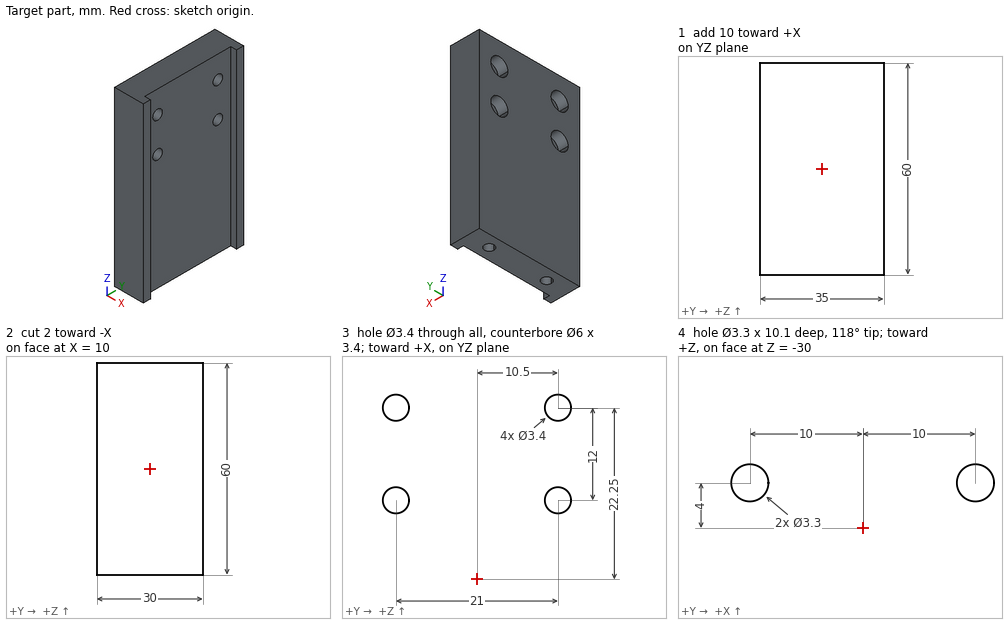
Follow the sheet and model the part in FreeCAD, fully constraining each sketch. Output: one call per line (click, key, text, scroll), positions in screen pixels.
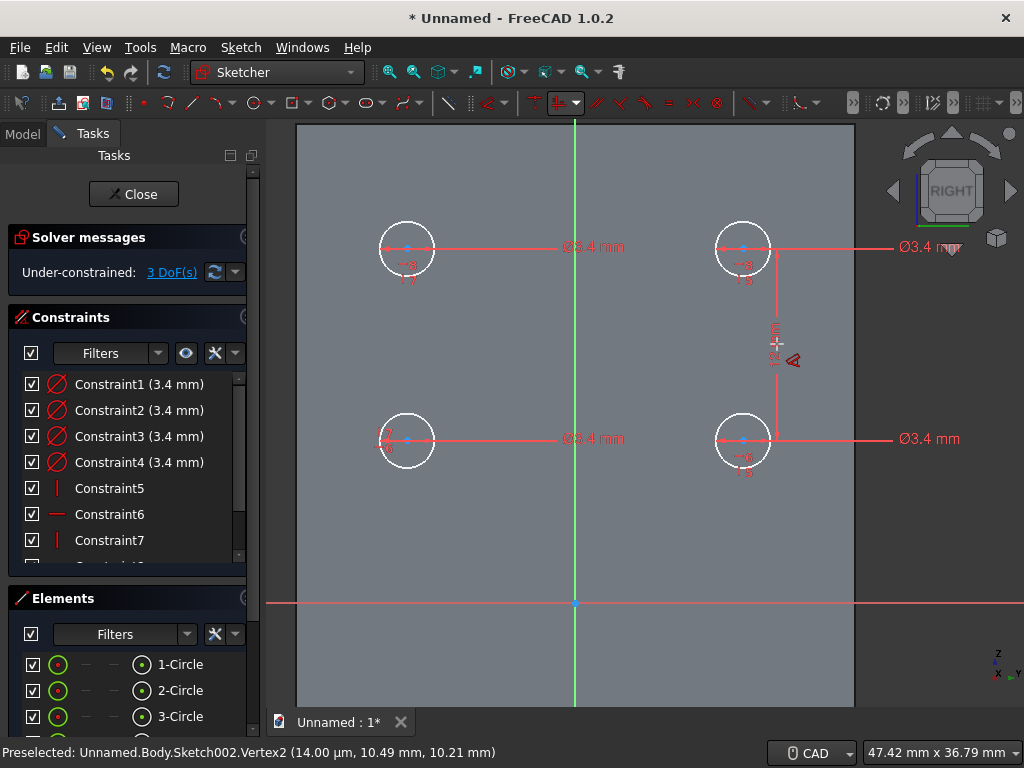
click(743, 441)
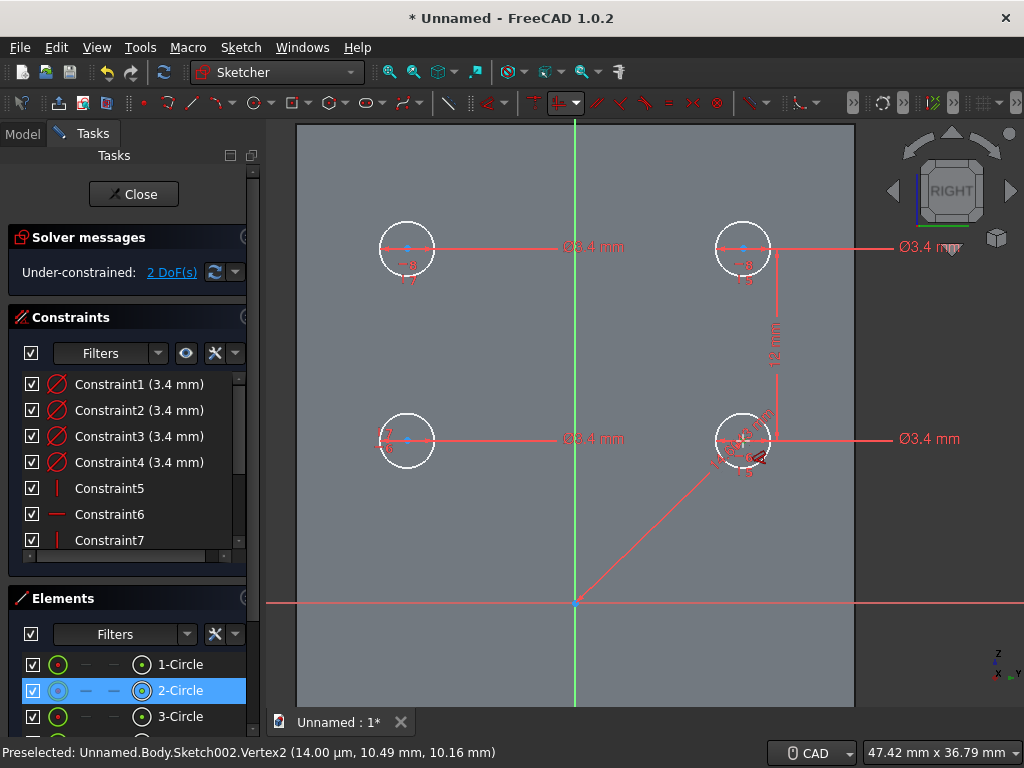
click(407, 441)
click(498, 475)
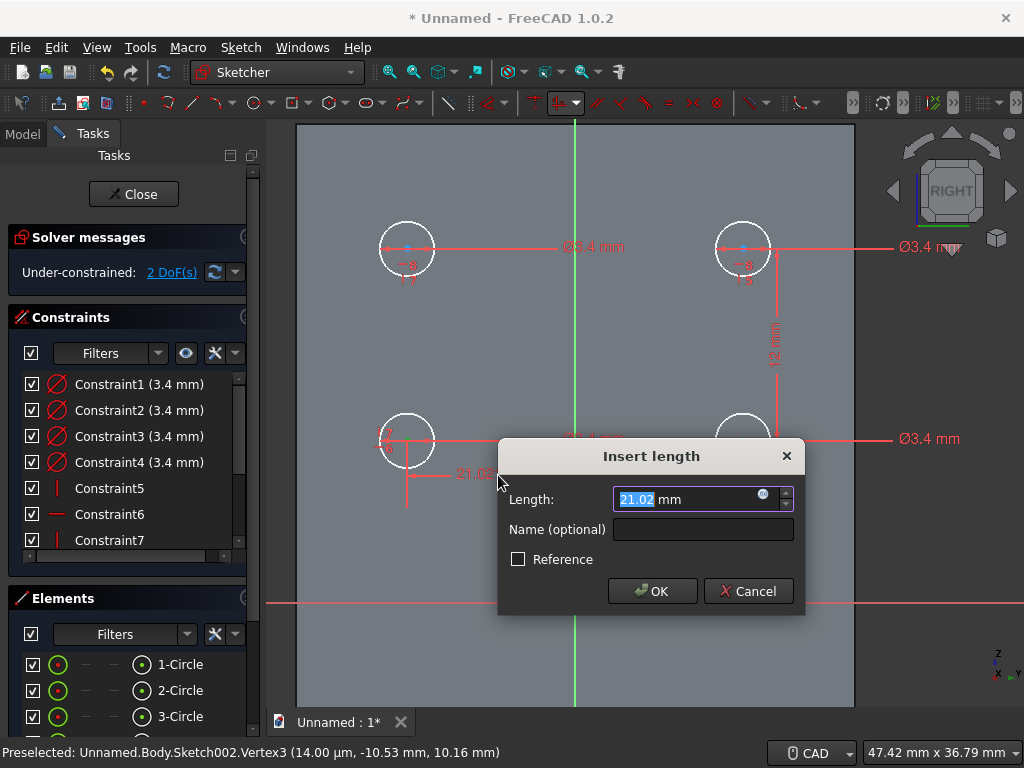
text(21)
key(Return)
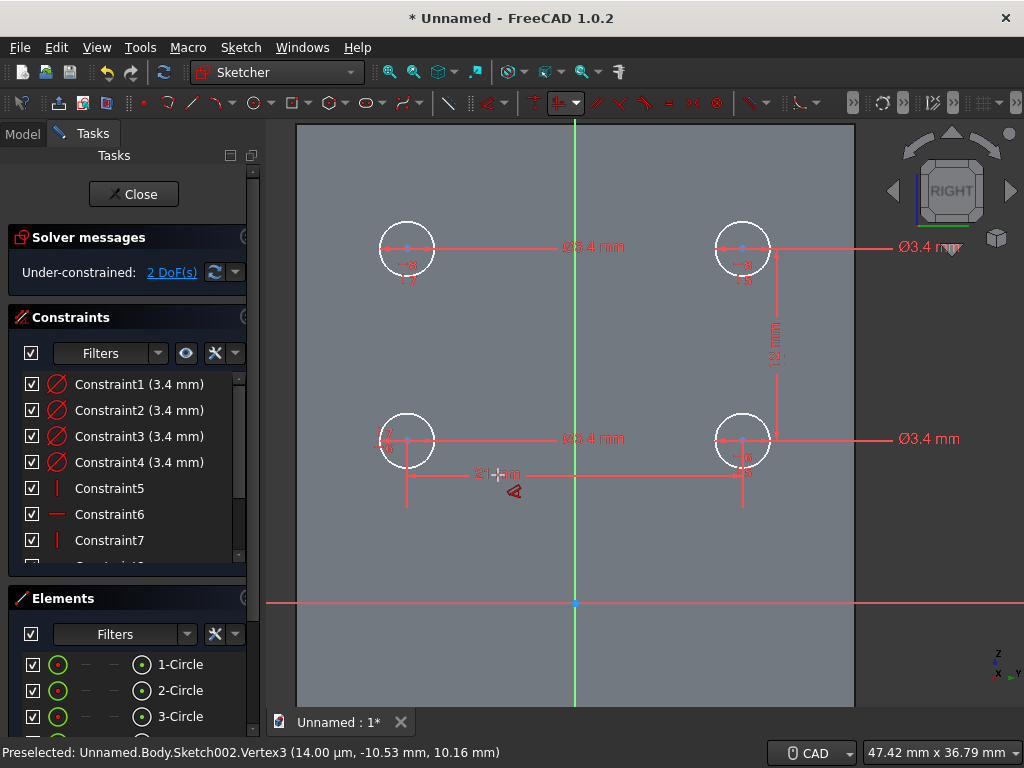
click(743, 249)
click(659, 637)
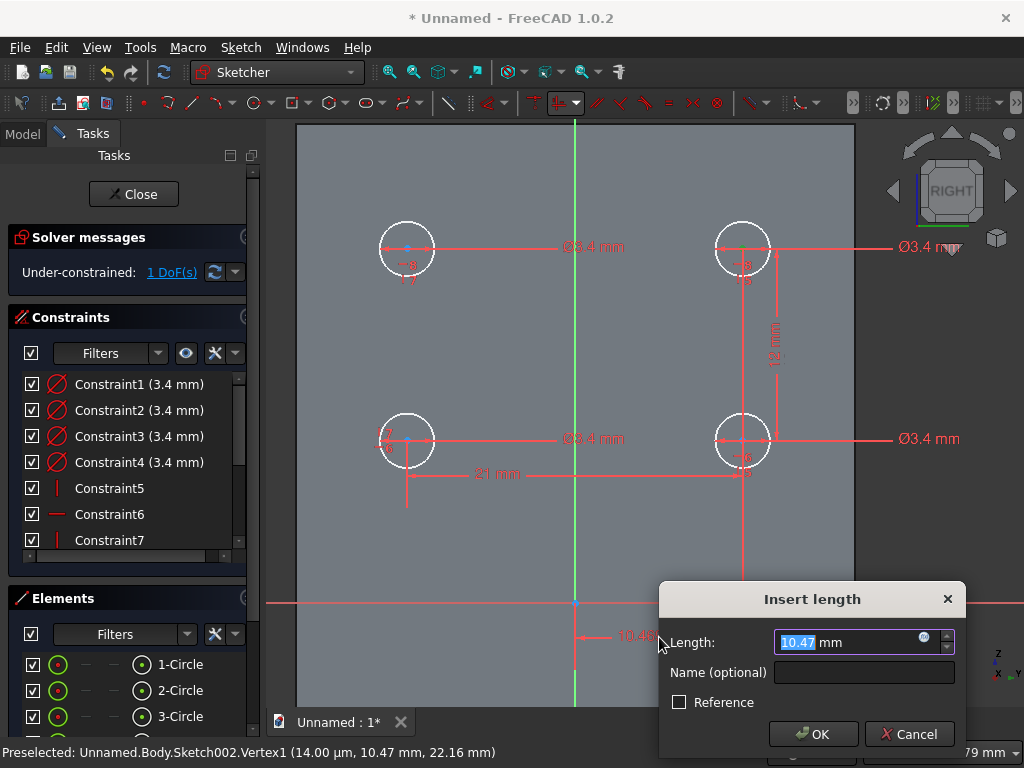
text(10.5)
key(Return)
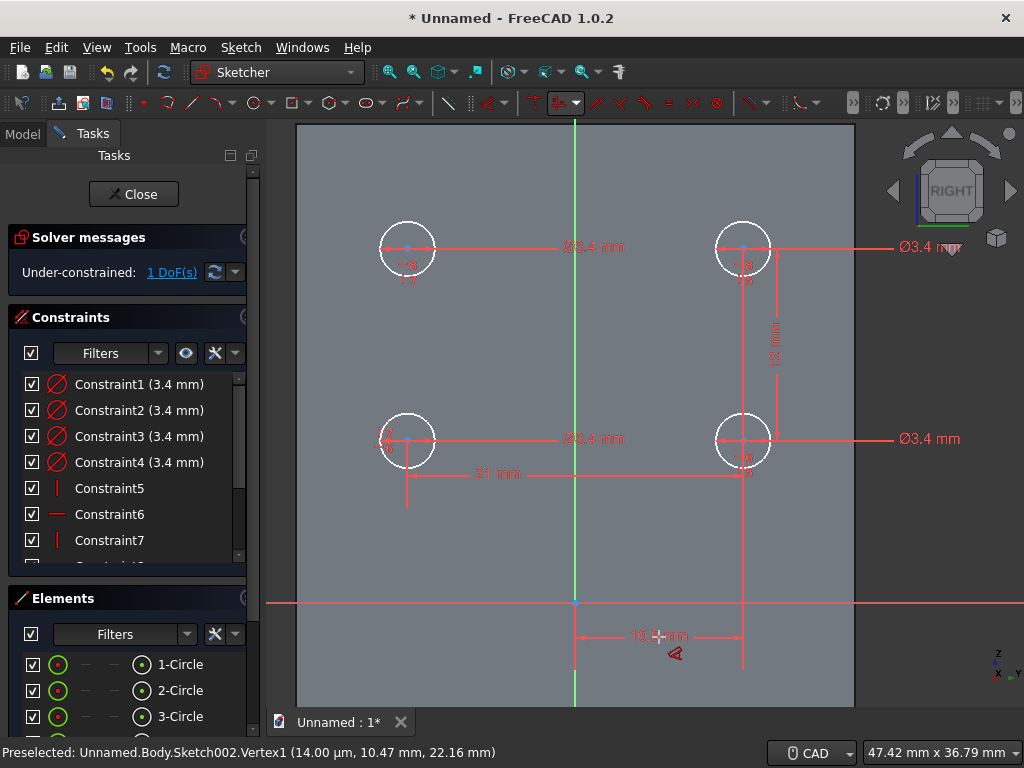
click(743, 249)
click(777, 508)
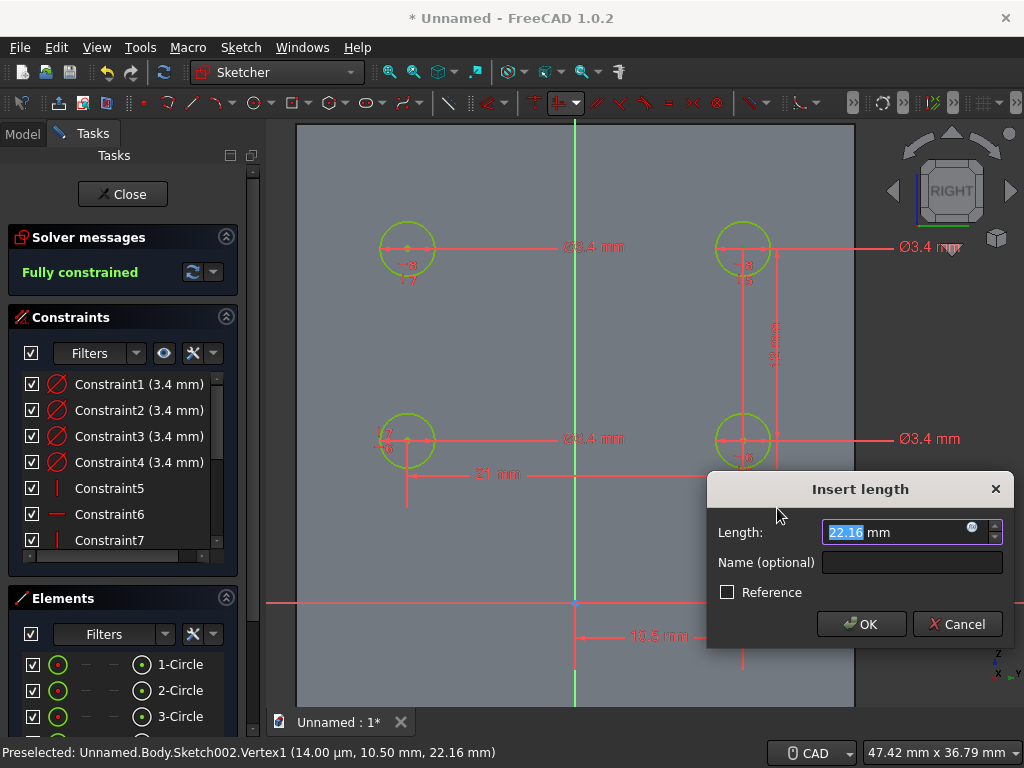
text(22.25)
key(Return)
key(Escape)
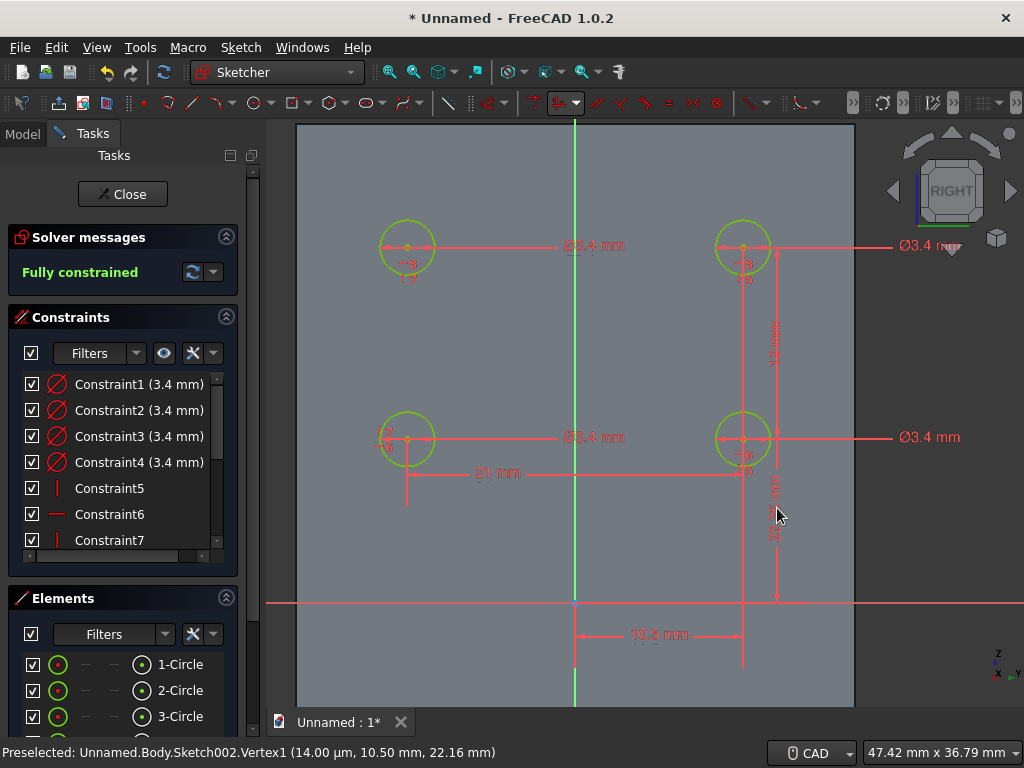
click(123, 194)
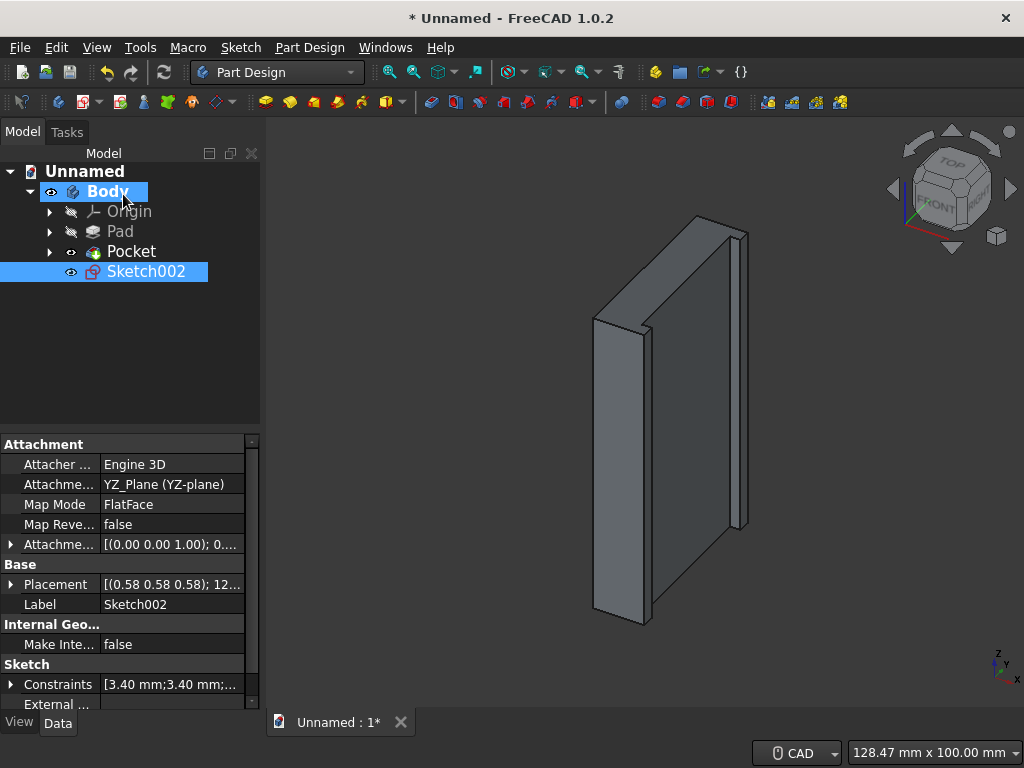
click(456, 102)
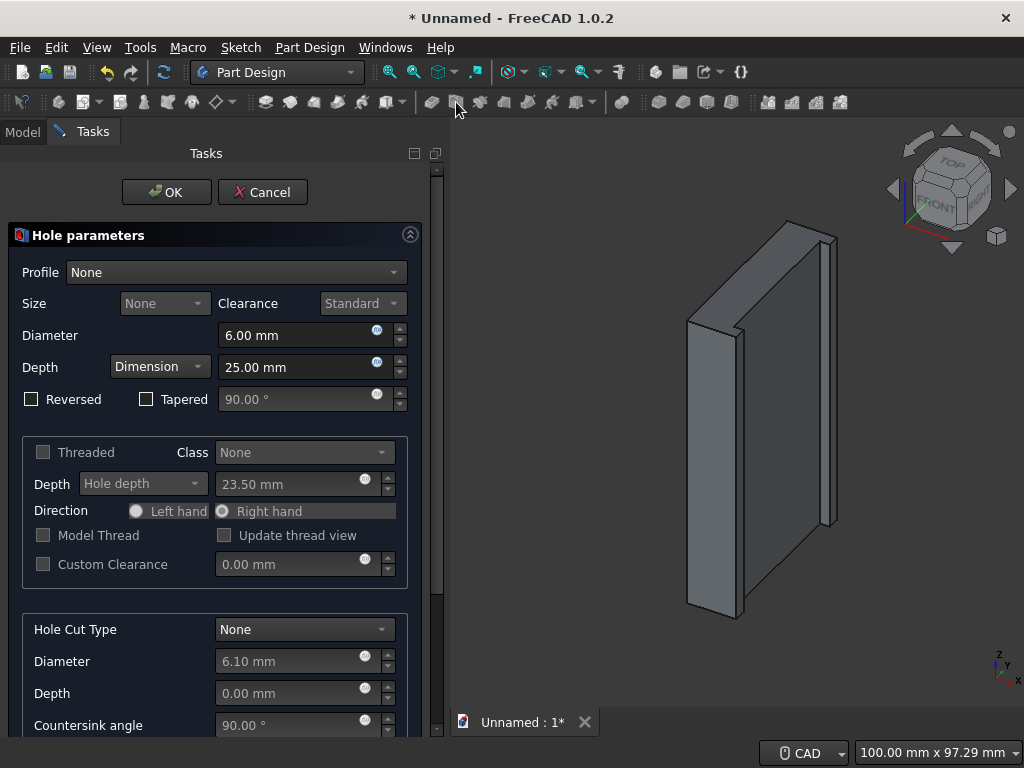
triple_click(305, 335)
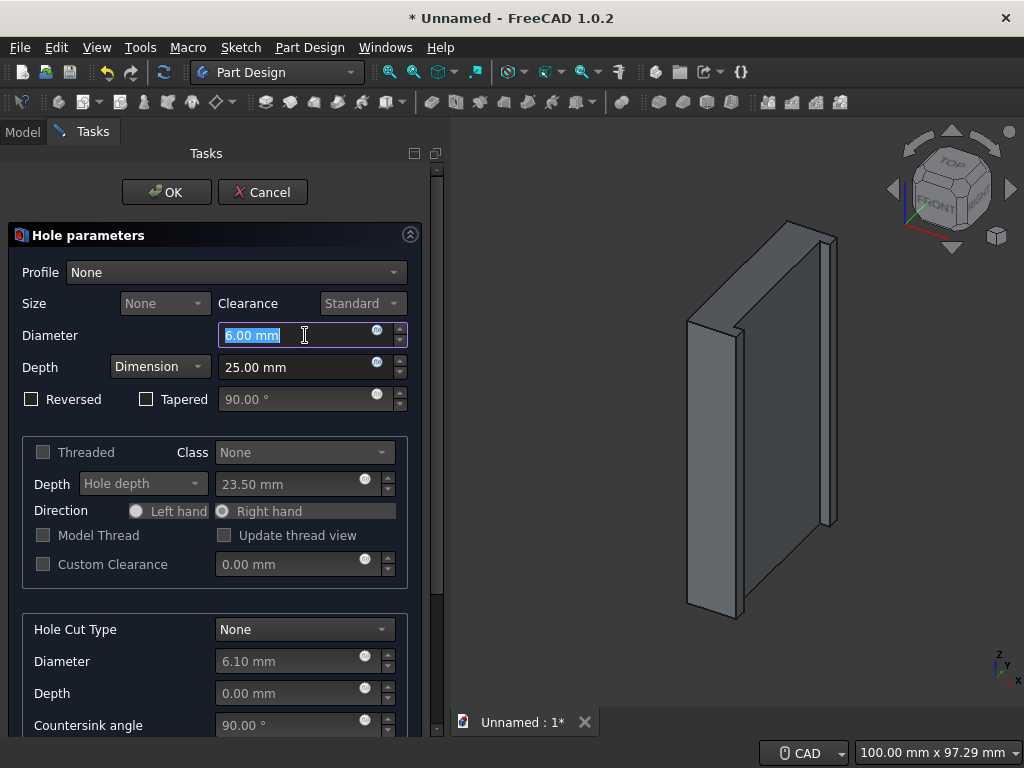
text(3.4)
key(Tab)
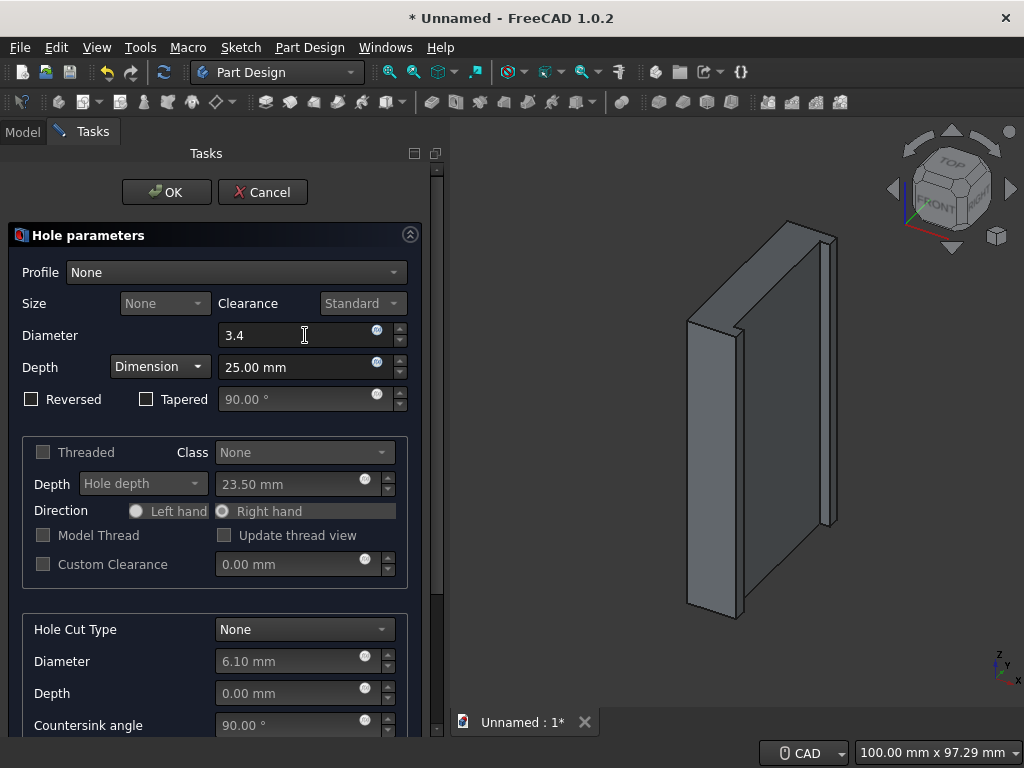
click(161, 366)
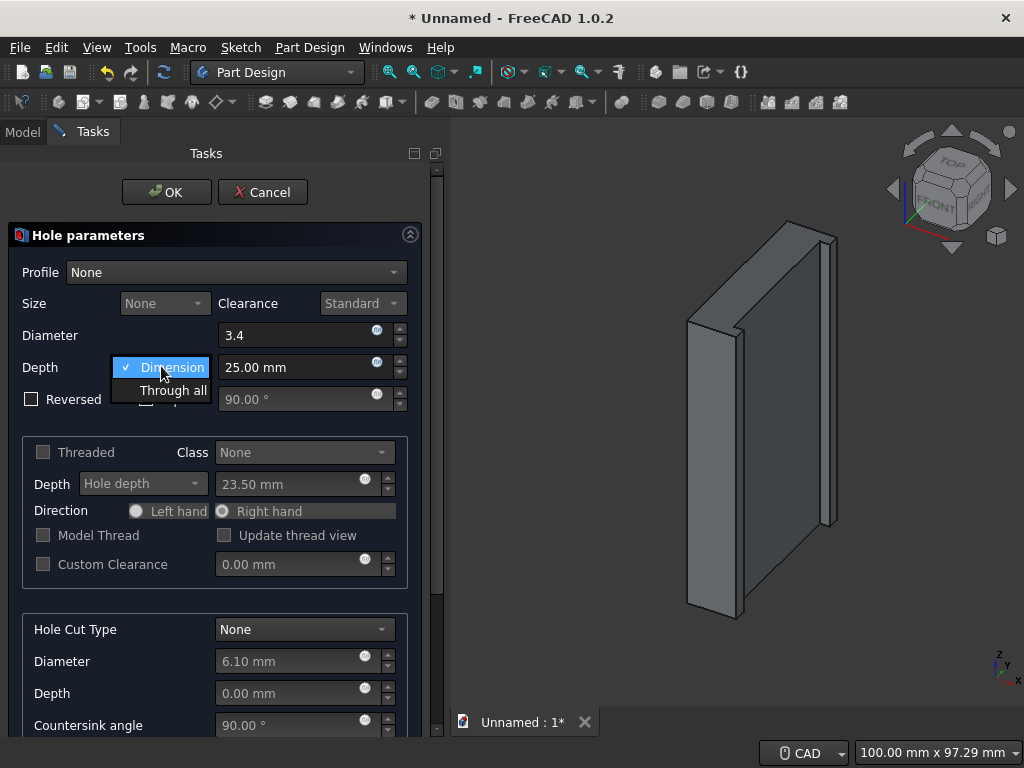
click(160, 390)